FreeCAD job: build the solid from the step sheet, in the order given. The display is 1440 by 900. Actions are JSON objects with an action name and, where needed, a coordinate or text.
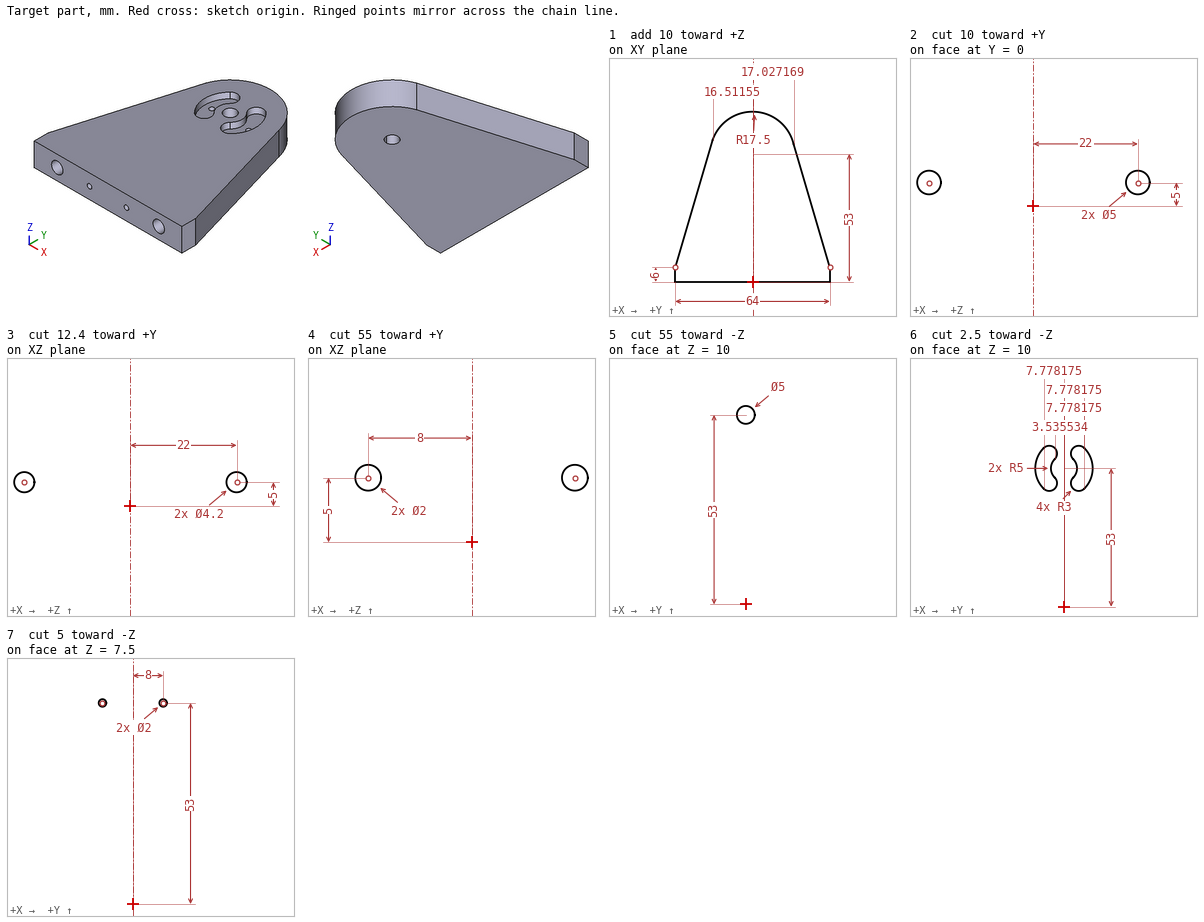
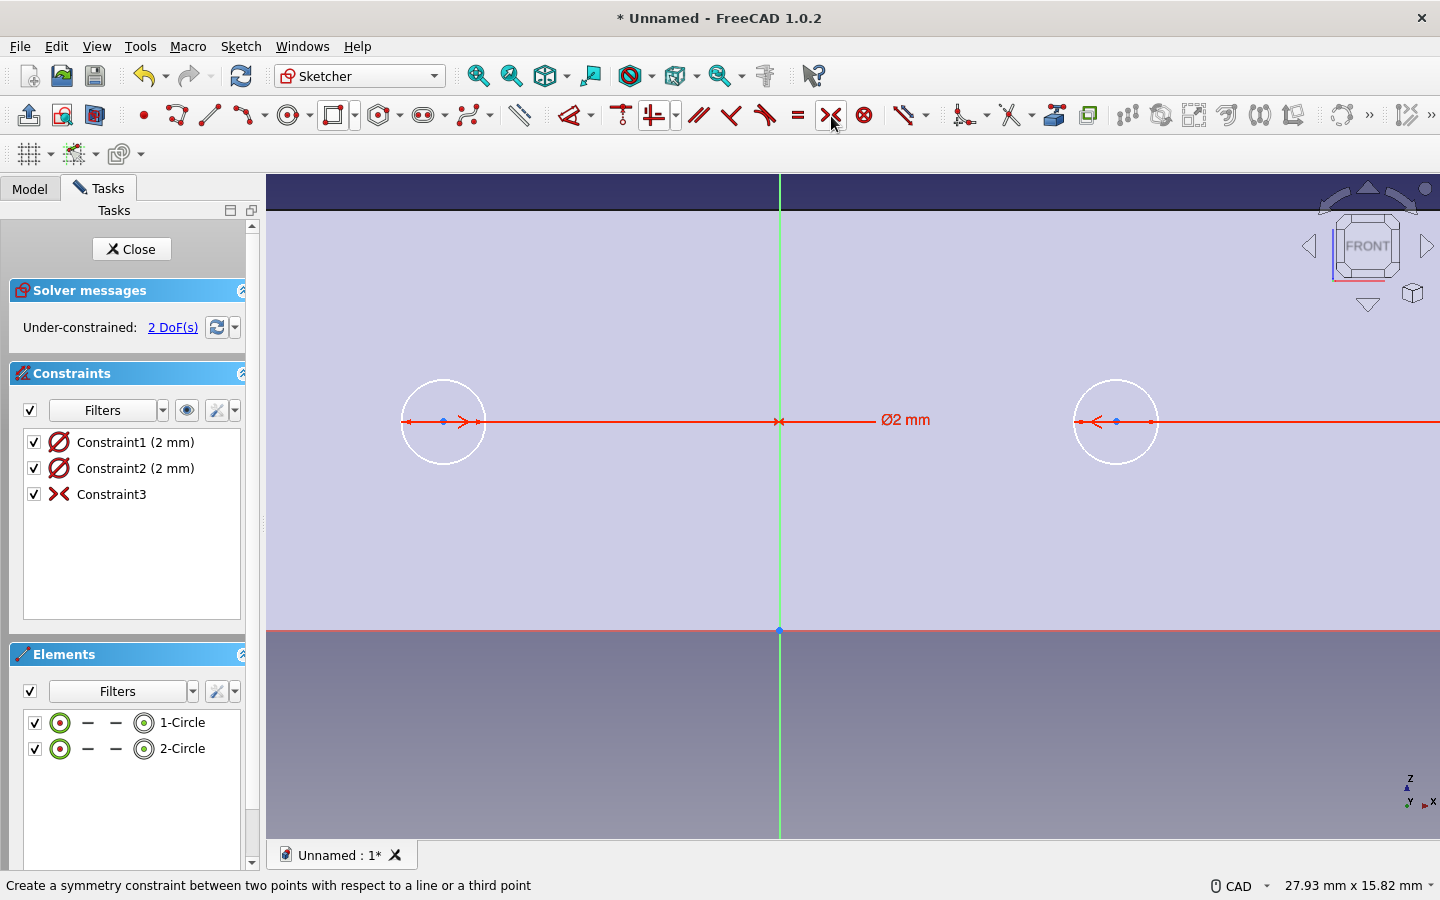
{"action": "left_click", "coordinate": [568, 116]}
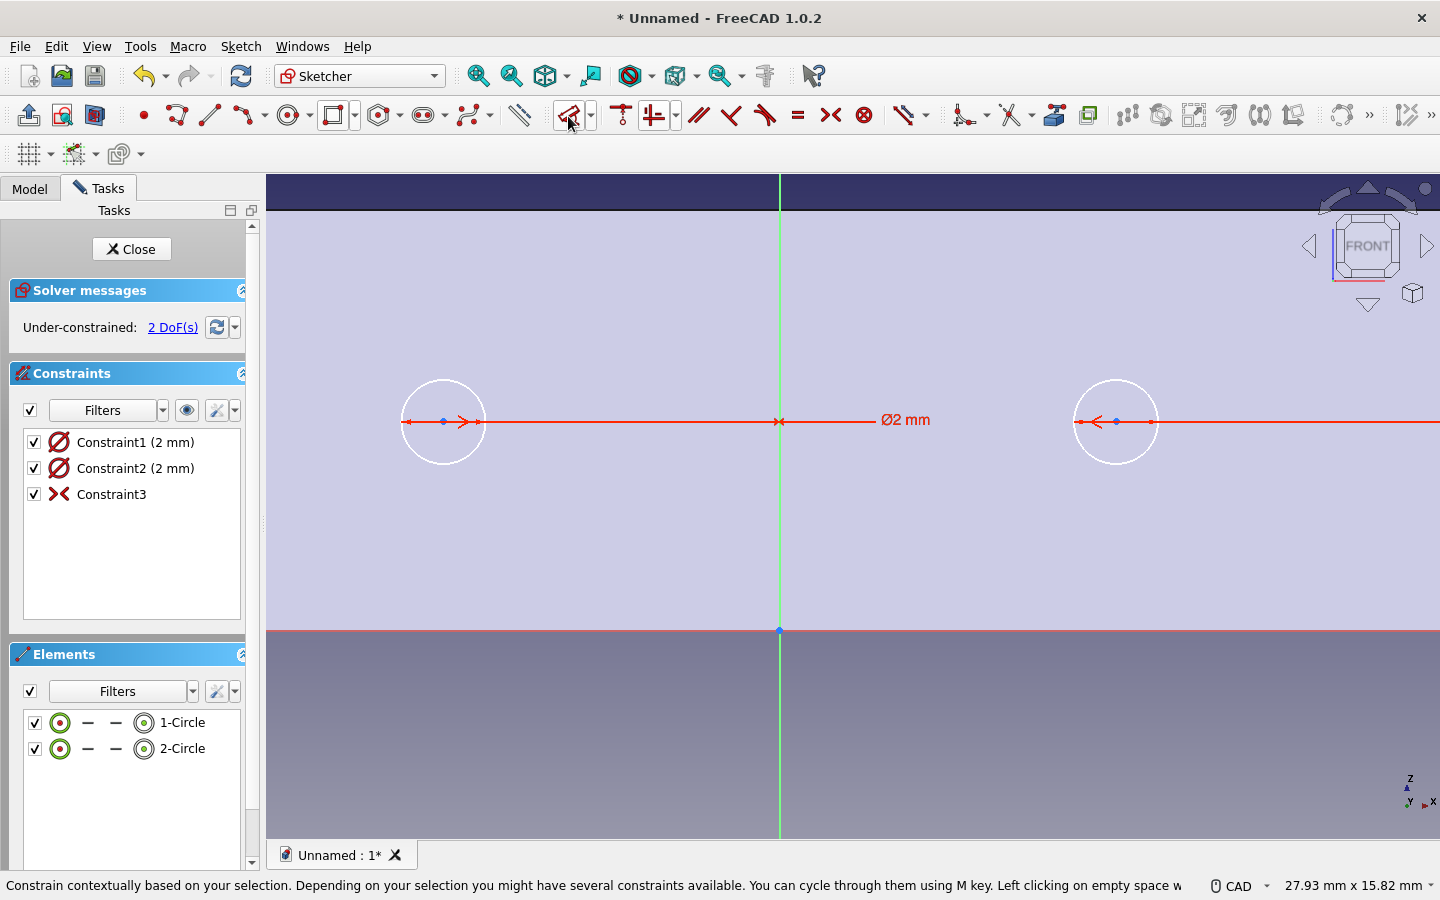
{"action": "left_click", "coordinate": [443, 422]}
{"action": "left_click", "coordinate": [612, 665]}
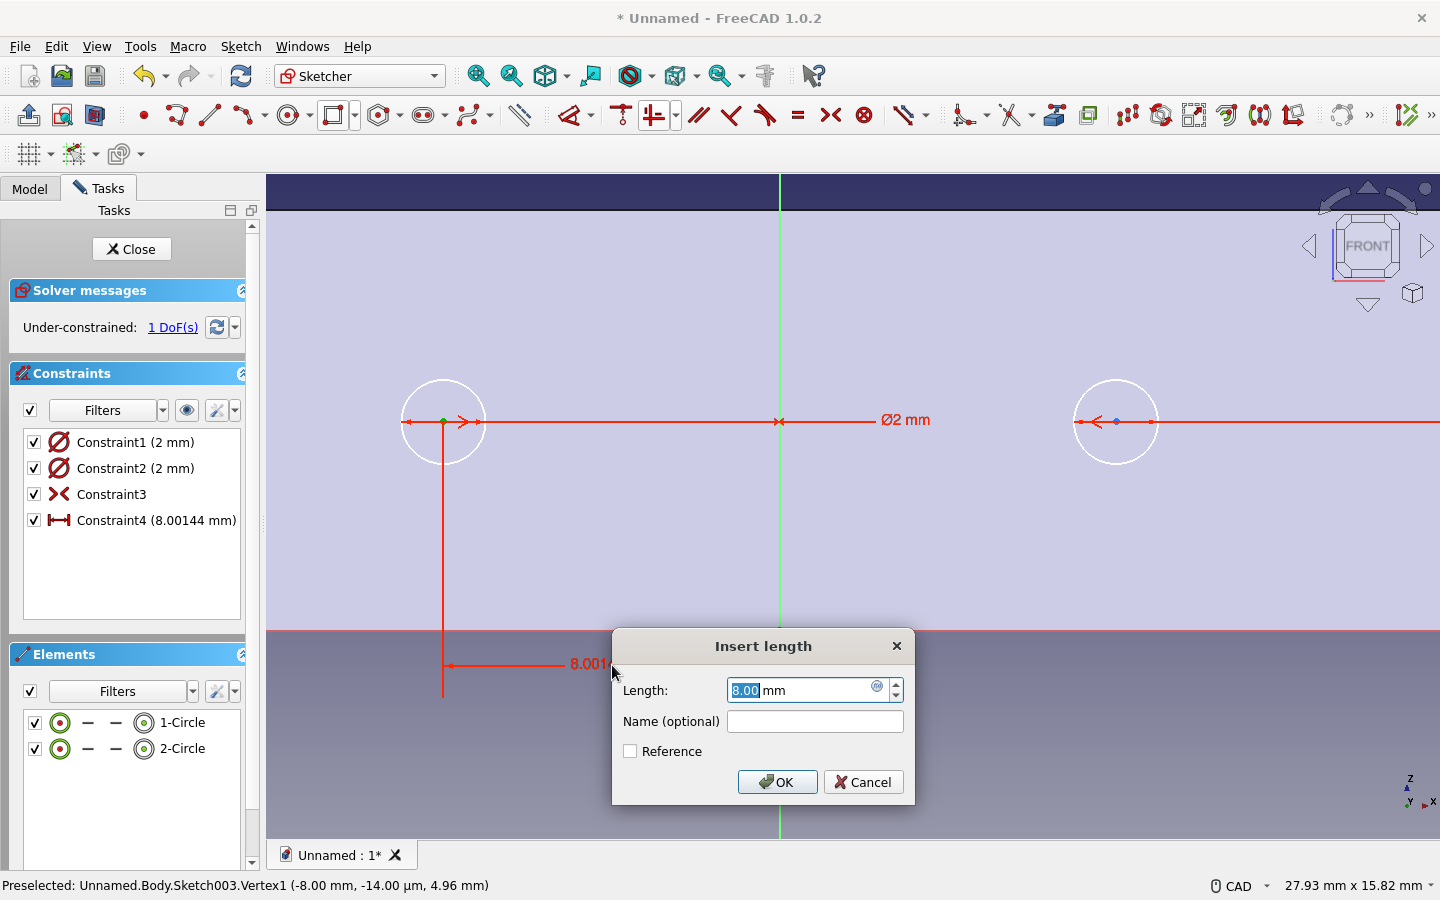
{"action": "type", "text": "8"}
{"action": "key", "text": "Return"}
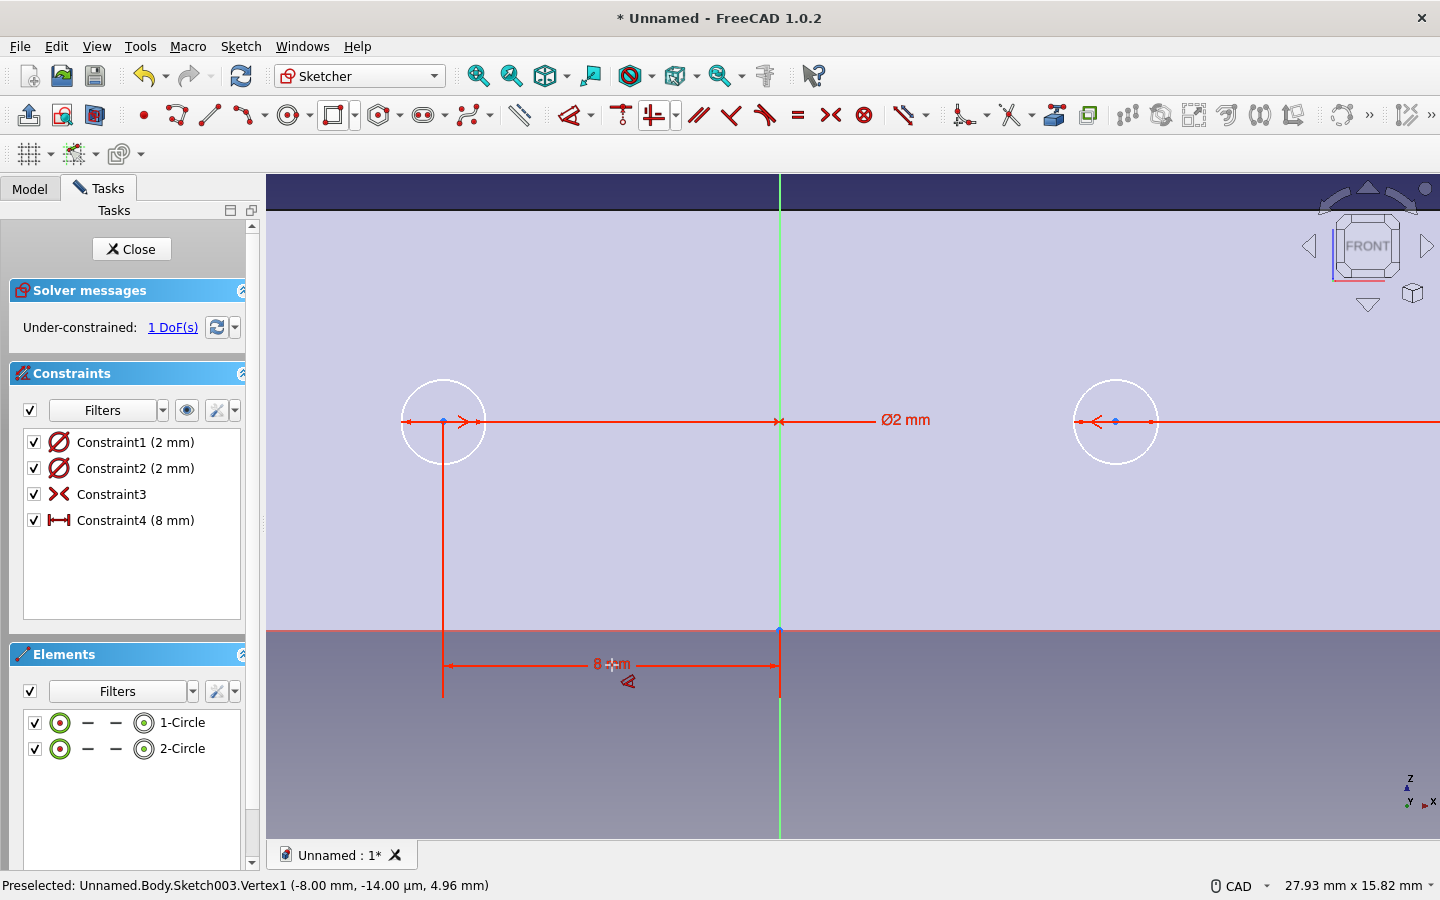
{"action": "left_click", "coordinate": [443, 422]}
{"action": "left_click", "coordinate": [409, 526]}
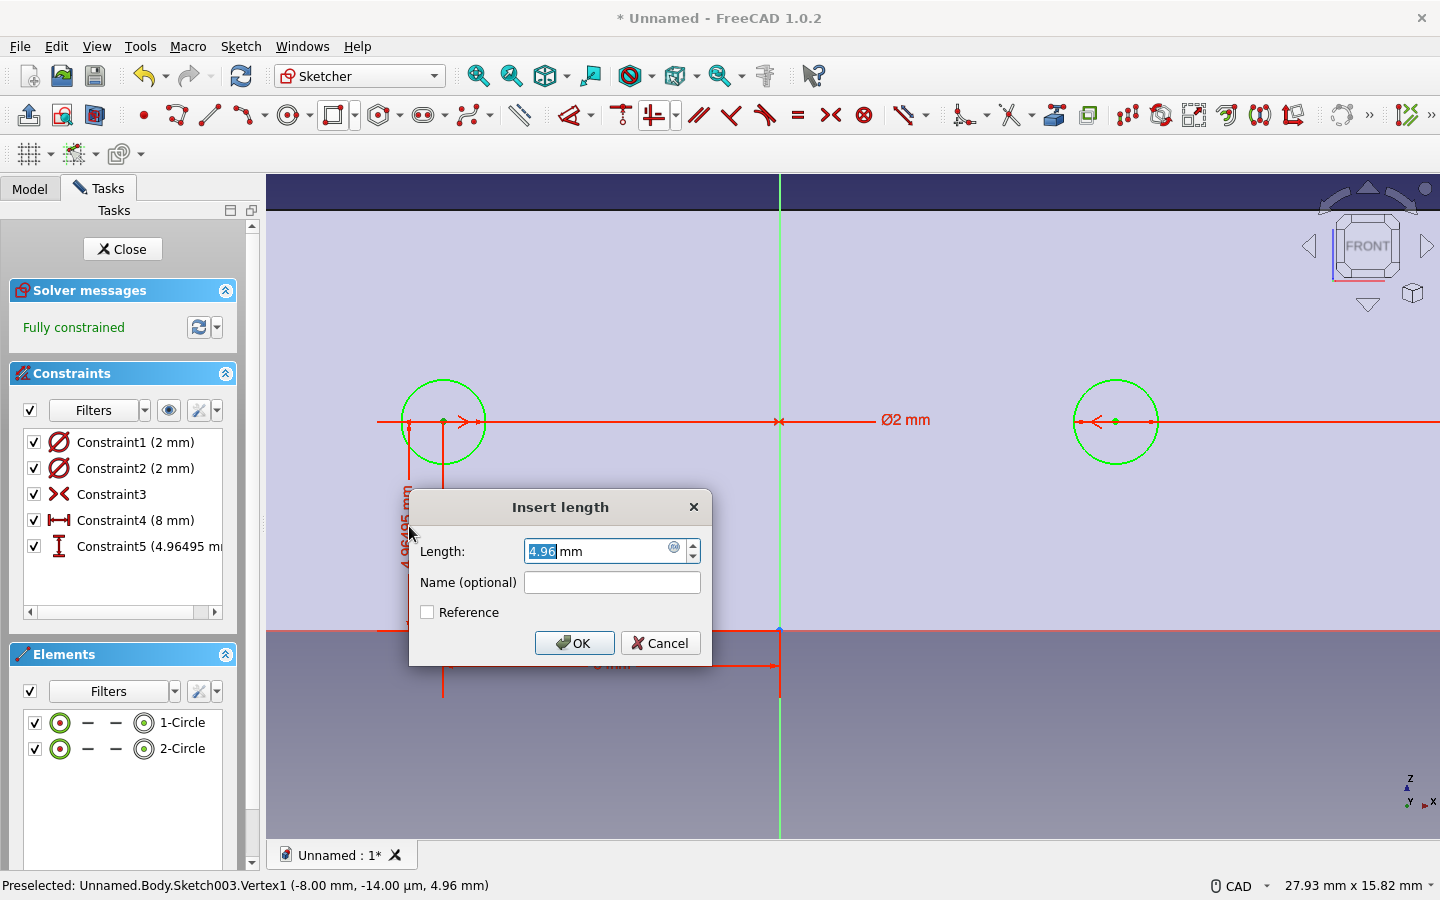
{"action": "type", "text": "5"}
{"action": "key", "text": "Return"}
{"action": "key", "text": "Escape"}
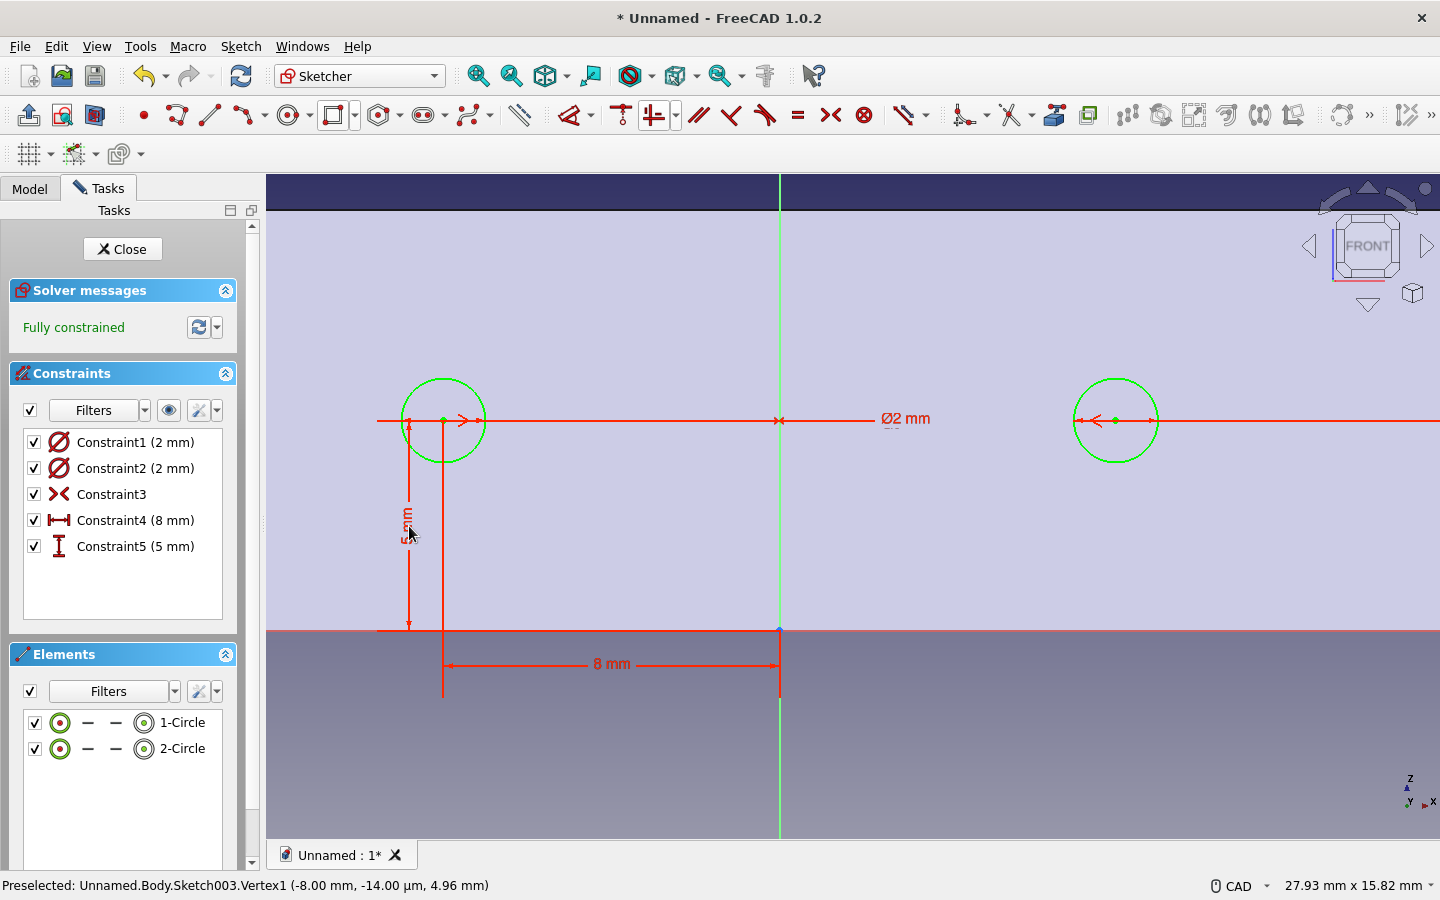
{"action": "left_click", "coordinate": [123, 249]}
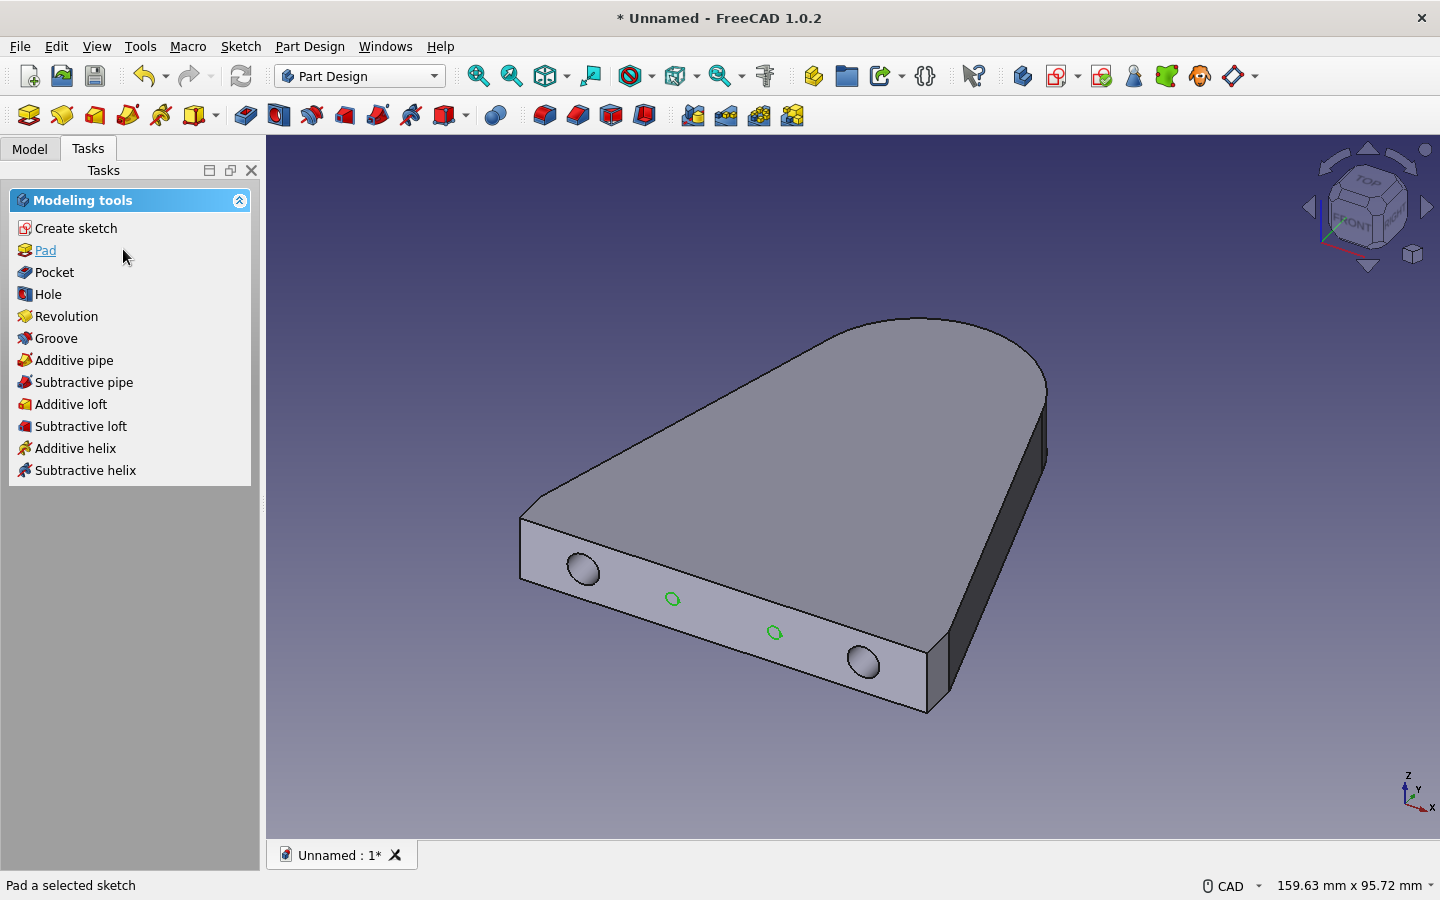
{"action": "left_click", "coordinate": [246, 116]}